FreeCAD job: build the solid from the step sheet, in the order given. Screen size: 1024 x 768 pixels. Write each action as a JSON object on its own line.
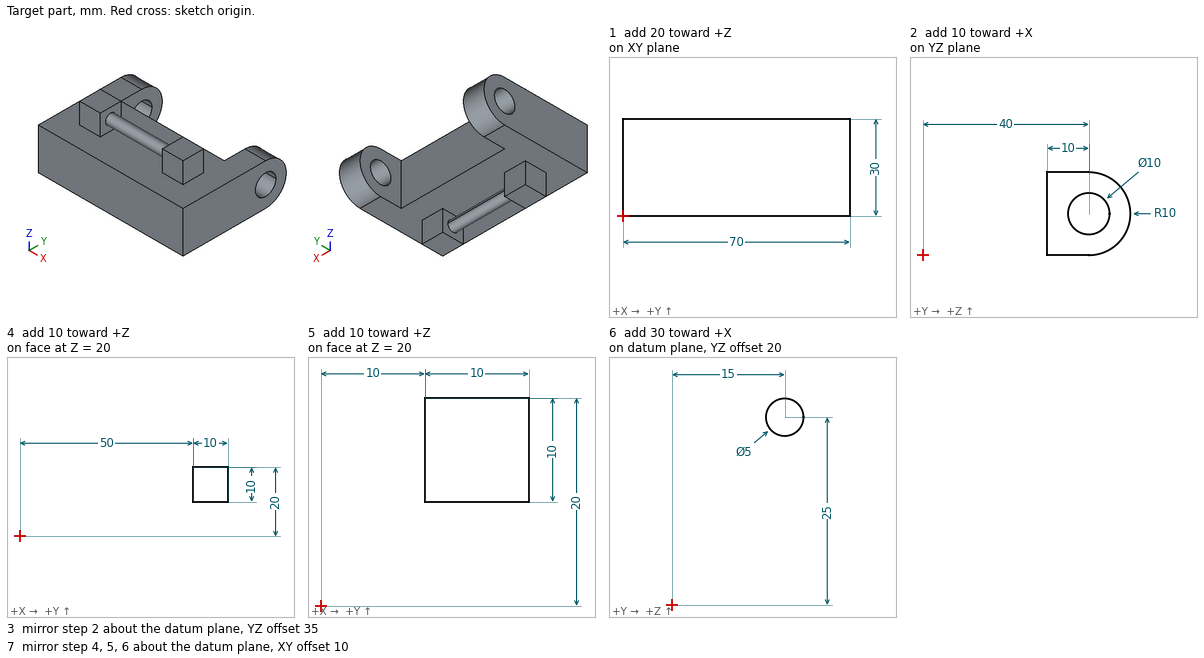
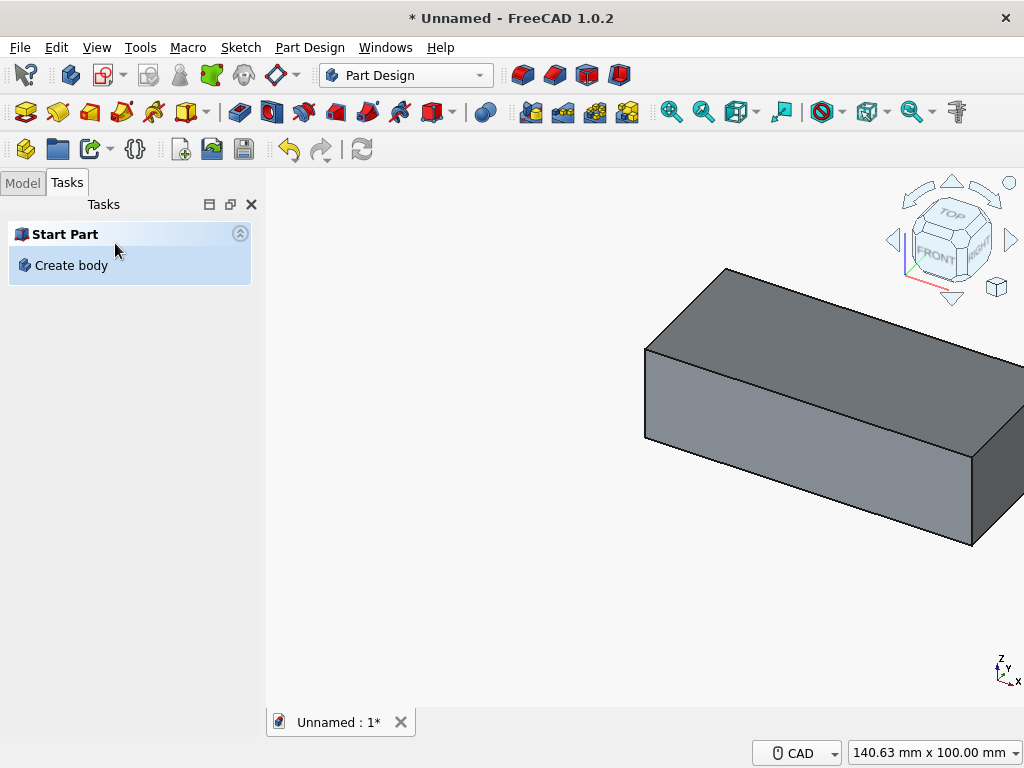
{"action": "key", "text": "v f"}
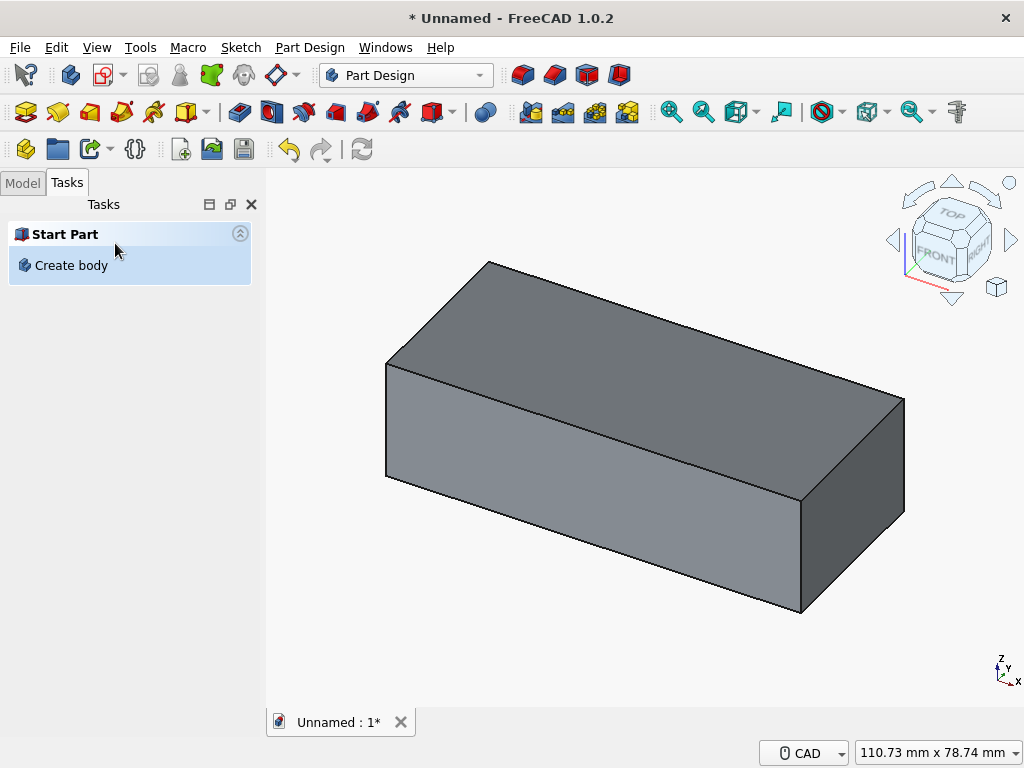
{"action": "left_click", "coordinate": [104, 76]}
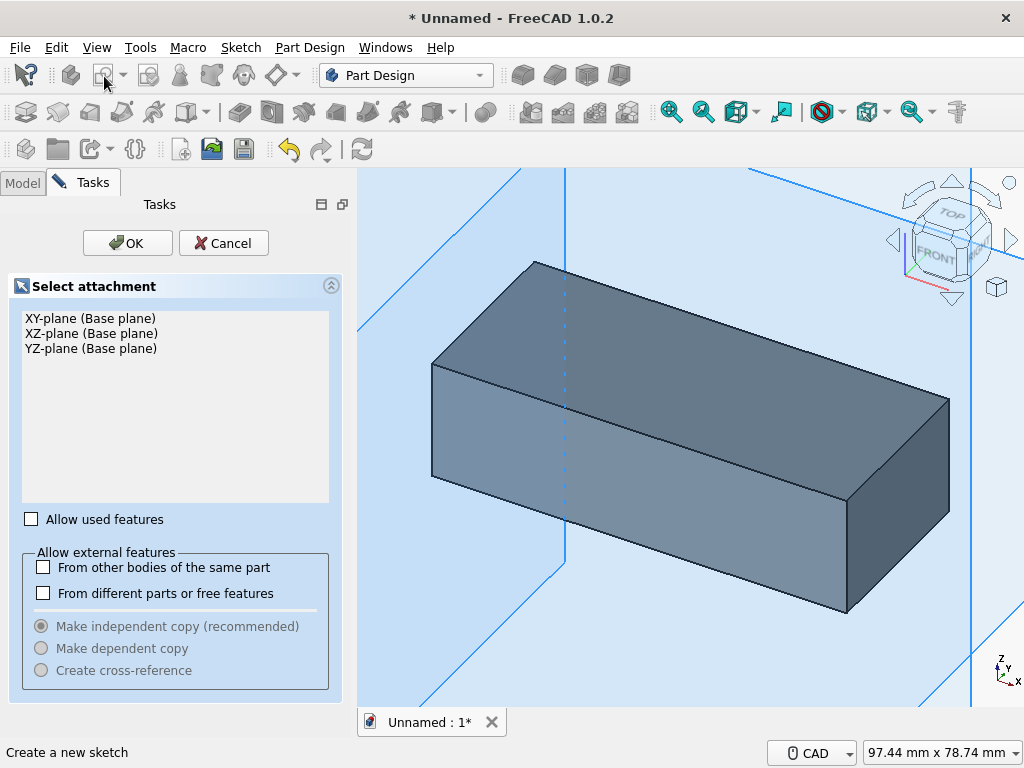
{"action": "left_click", "coordinate": [82, 348]}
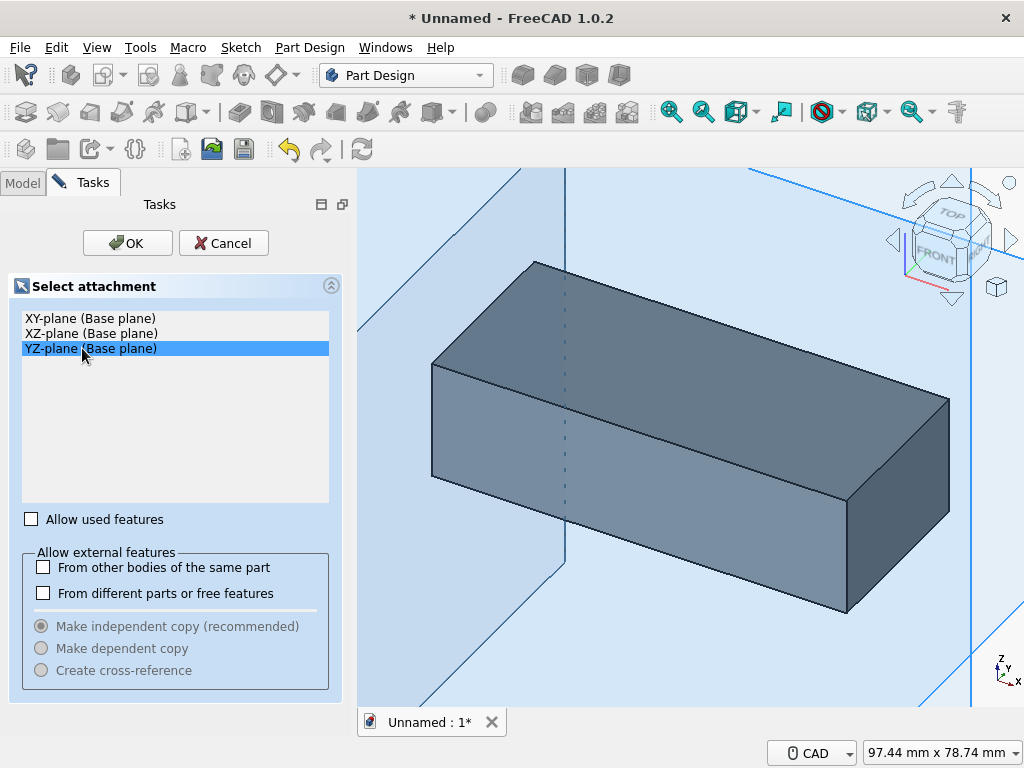
{"action": "left_click", "coordinate": [128, 243]}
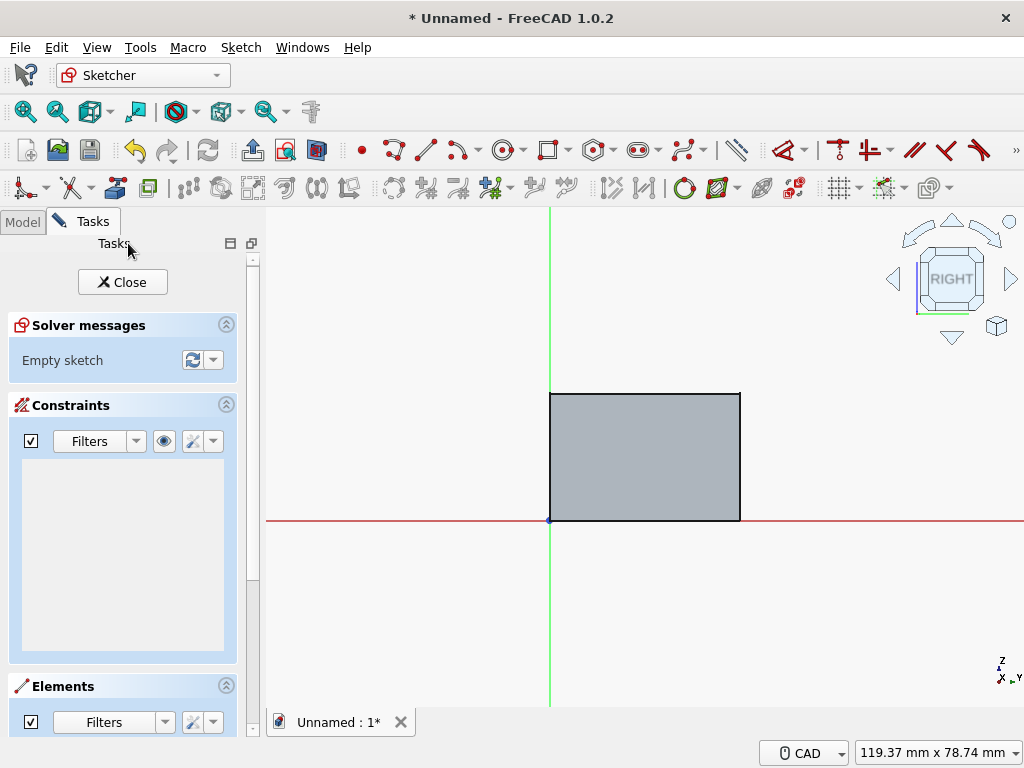
{"action": "key", "text": "q s"}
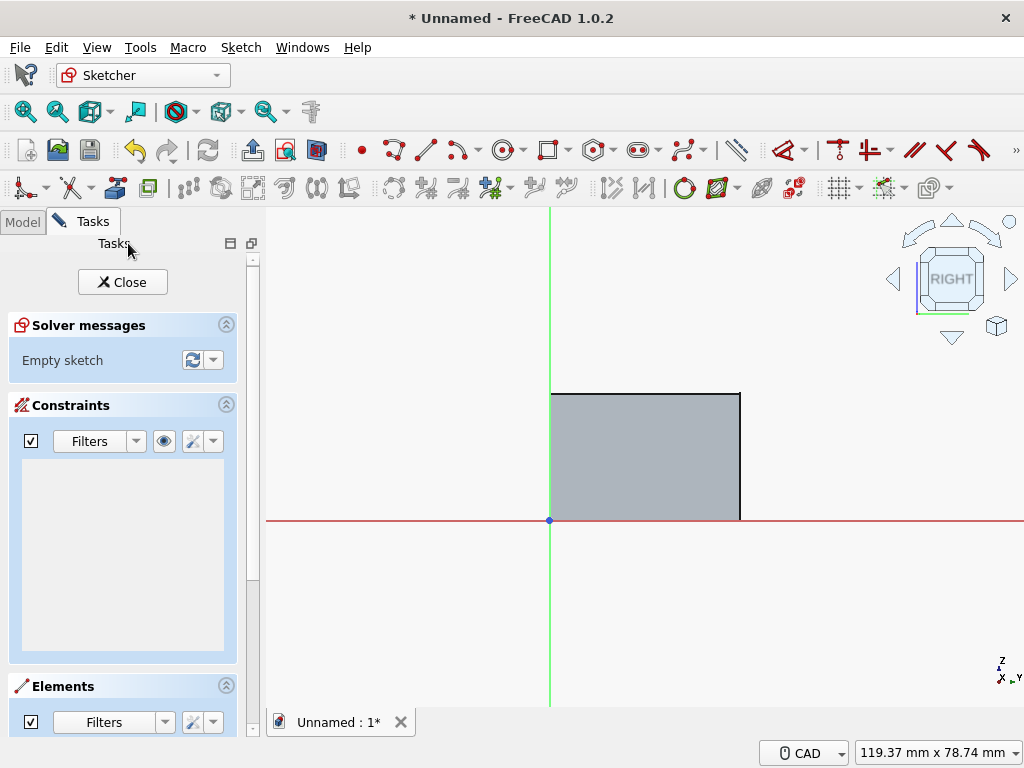
{"action": "scroll", "coordinate": [576, 457], "scroll_direction": "down", "scroll_amount": 5}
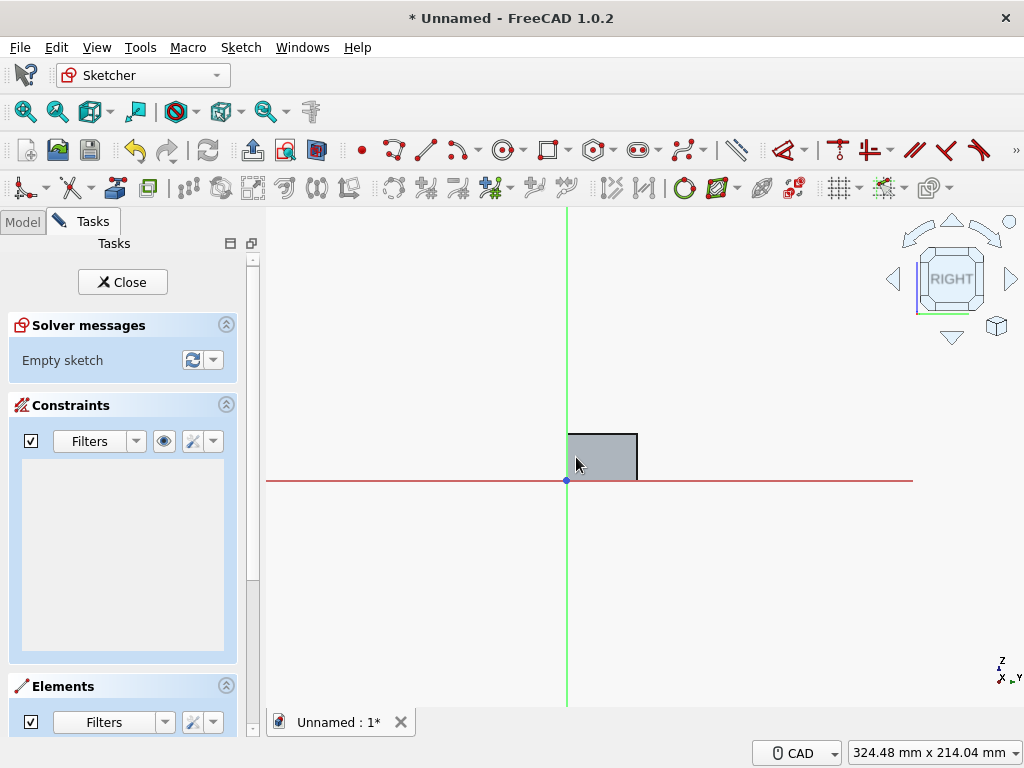
{"action": "scroll", "coordinate": [673, 457], "scroll_direction": "up", "scroll_amount": 10}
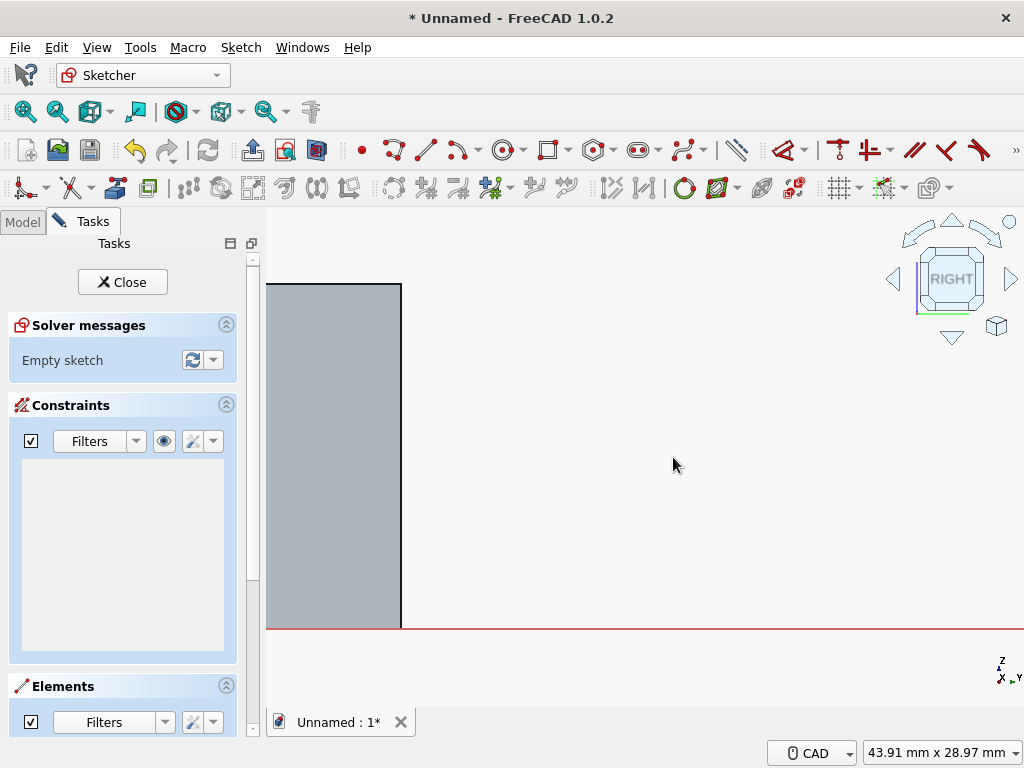
{"action": "key", "text": "g m"}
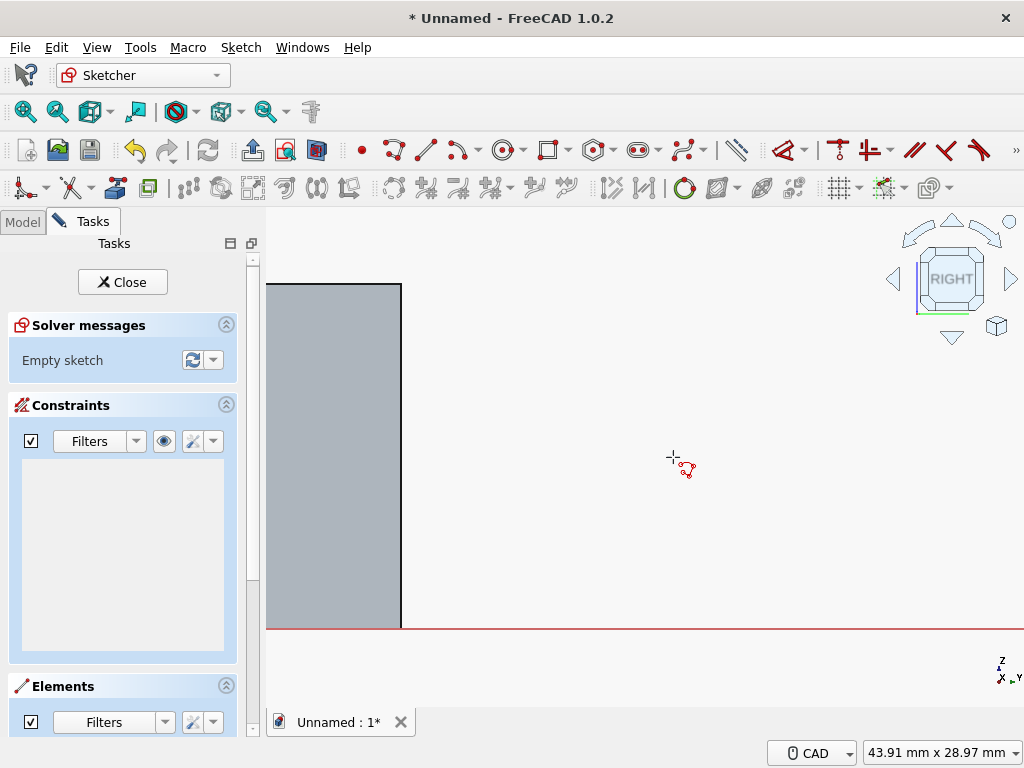
{"action": "left_click", "coordinate": [574, 284]}
{"action": "left_click", "coordinate": [401, 284]}
{"action": "left_click", "coordinate": [401, 629]}
{"action": "left_click", "coordinate": [574, 620]}
{"action": "right_click", "coordinate": [574, 620]}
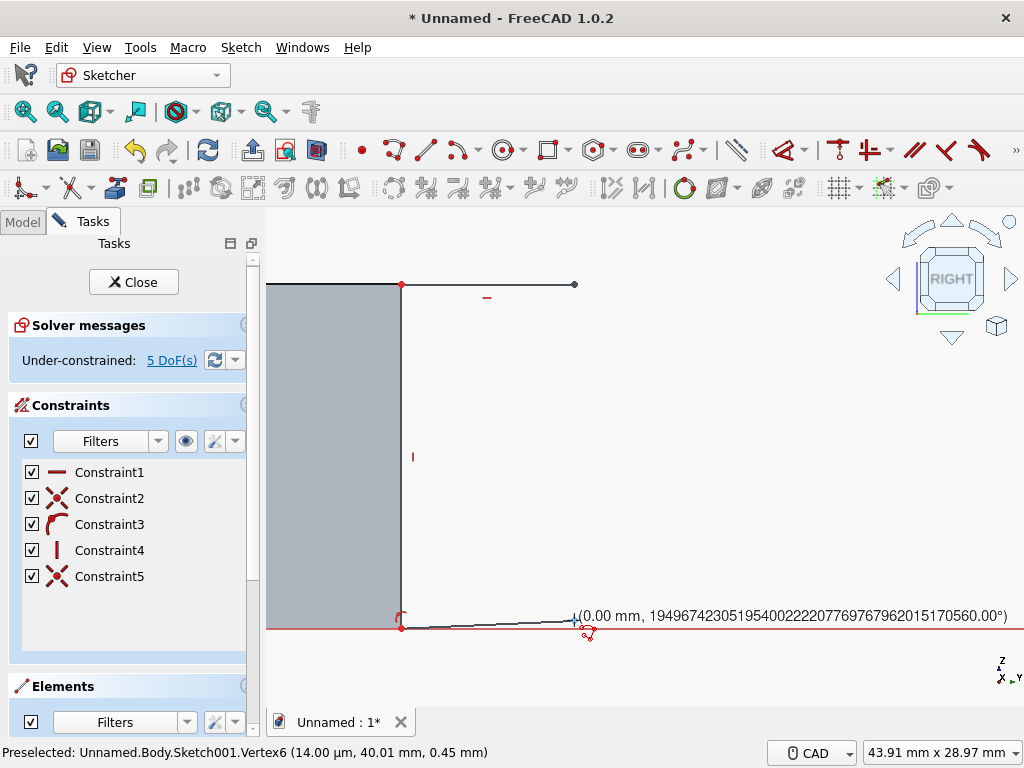
{"action": "key", "text": "g 3 a"}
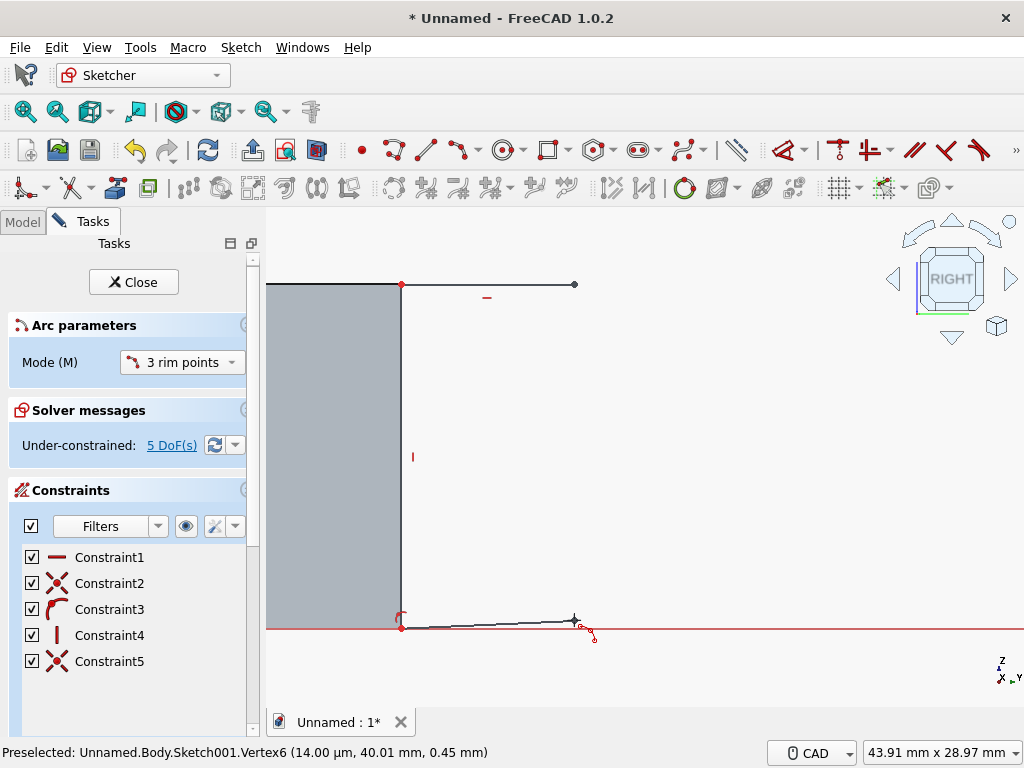
{"action": "left_click", "coordinate": [574, 621]}
{"action": "left_click", "coordinate": [574, 285]}
{"action": "left_click", "coordinate": [746, 456]}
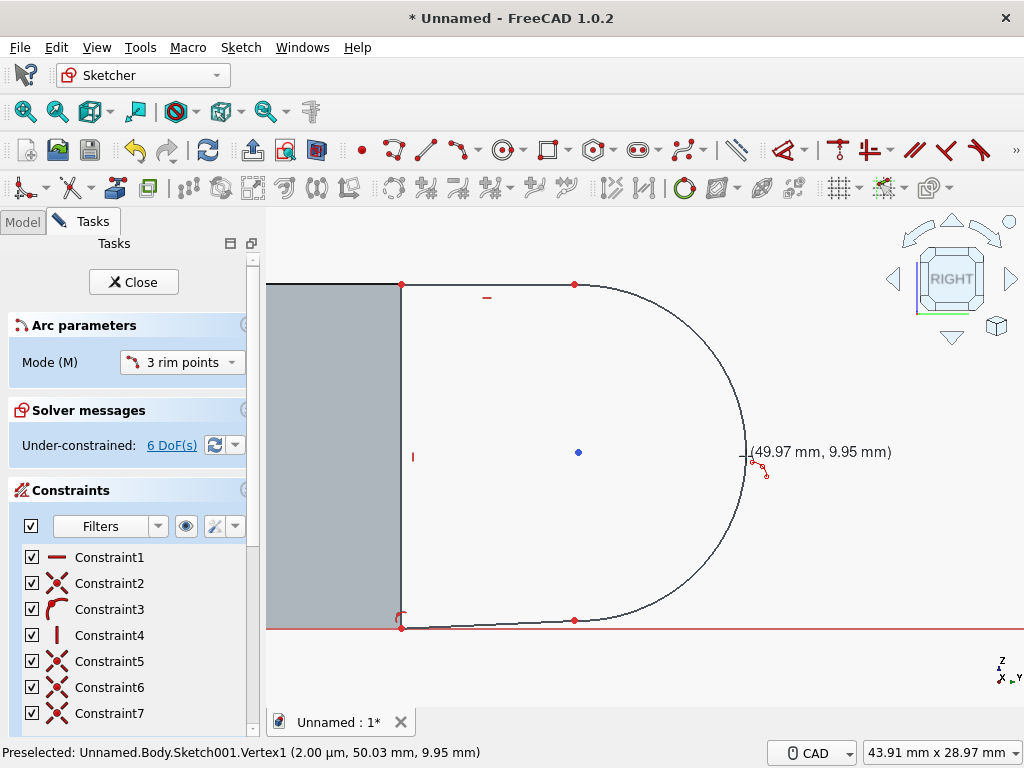
{"action": "key", "text": "g c"}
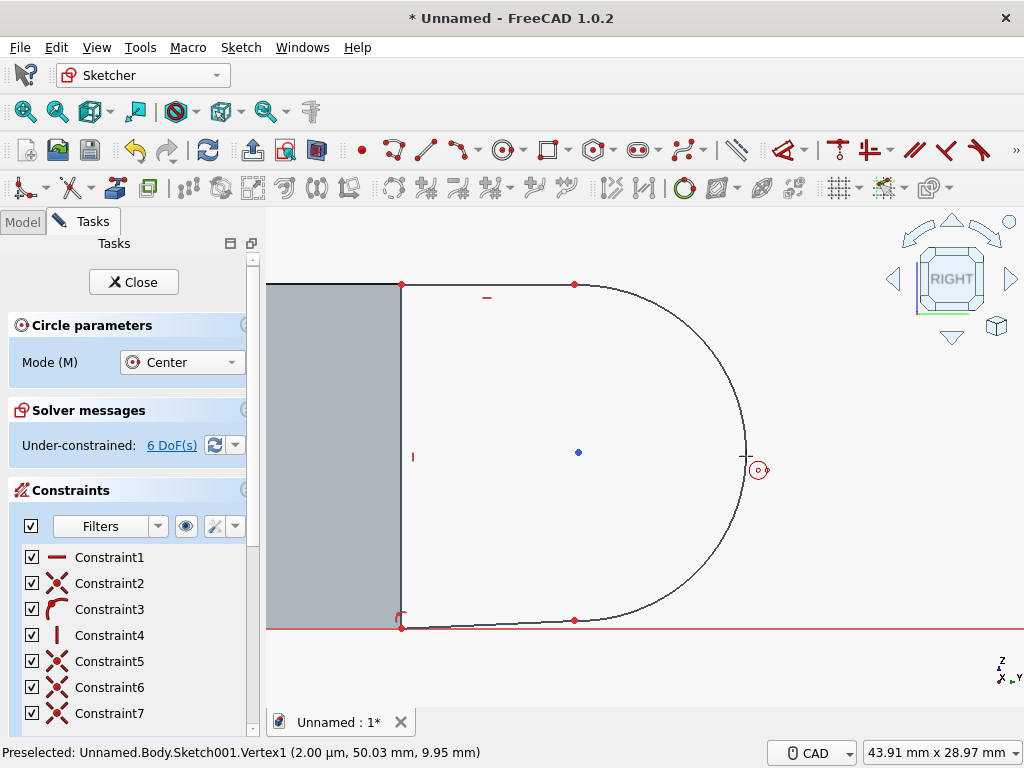
{"action": "left_click", "coordinate": [574, 456]}
{"action": "mouse_move", "coordinate": [635, 395]}